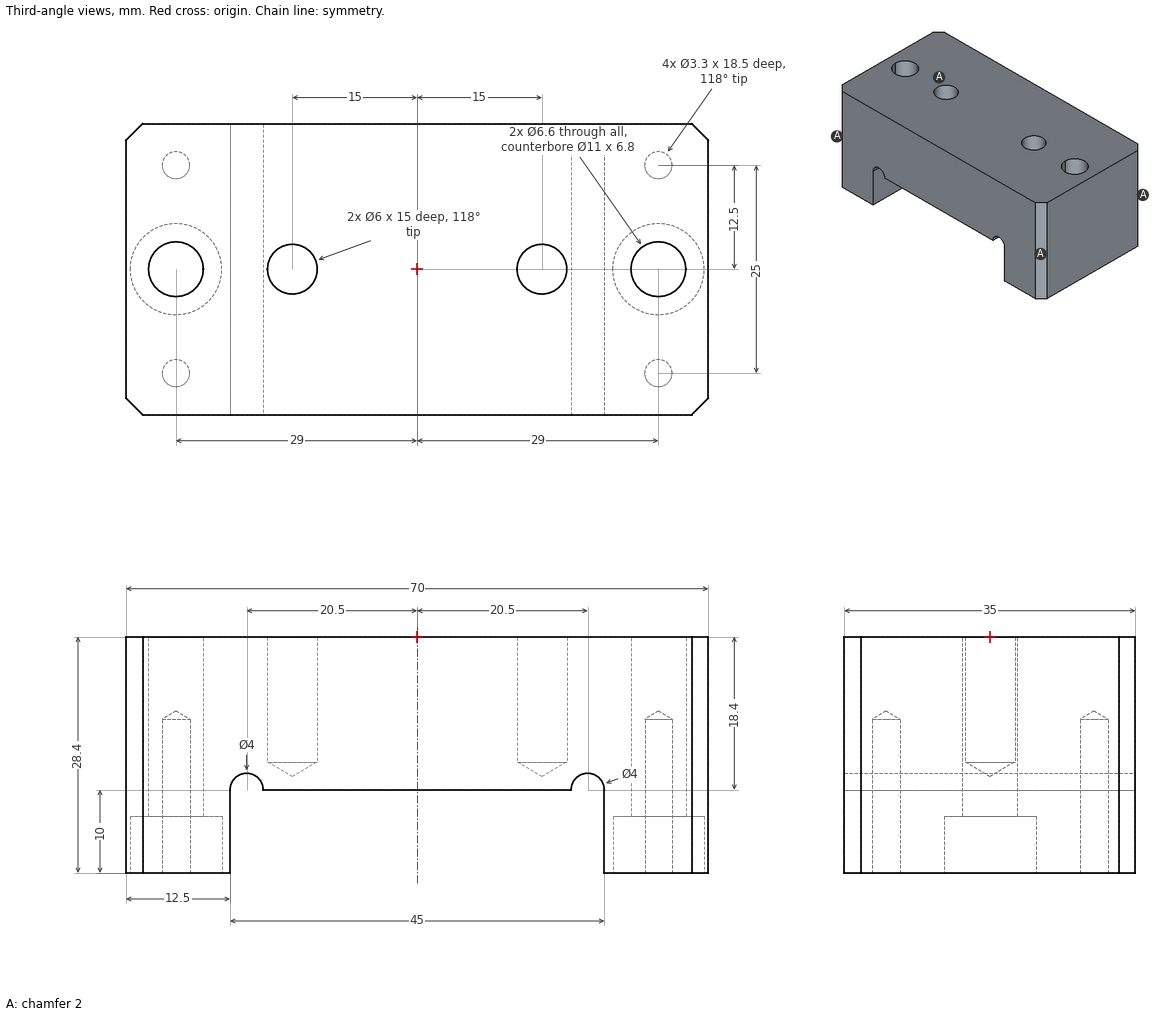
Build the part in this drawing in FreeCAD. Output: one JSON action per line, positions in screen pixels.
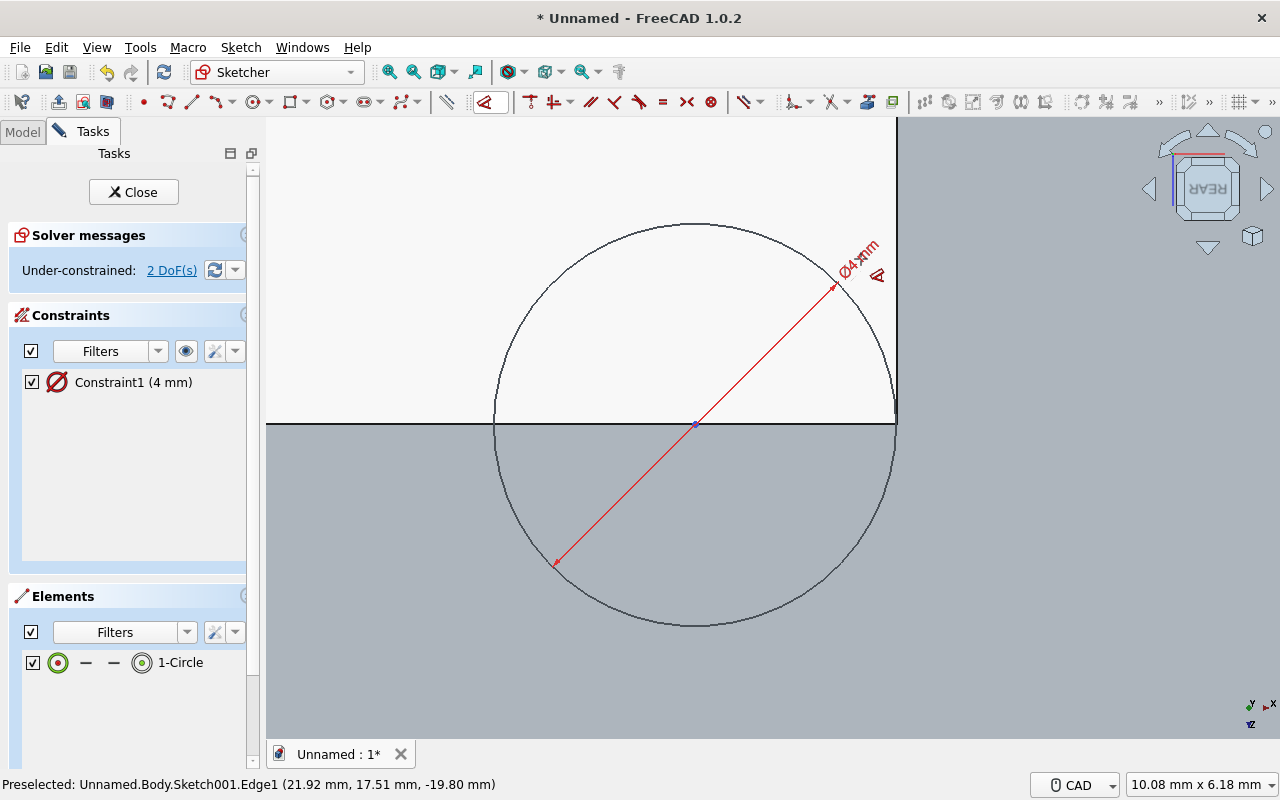
{"action": "left_click", "coordinate": [695, 425]}
{"action": "left_click", "coordinate": [402, 391]}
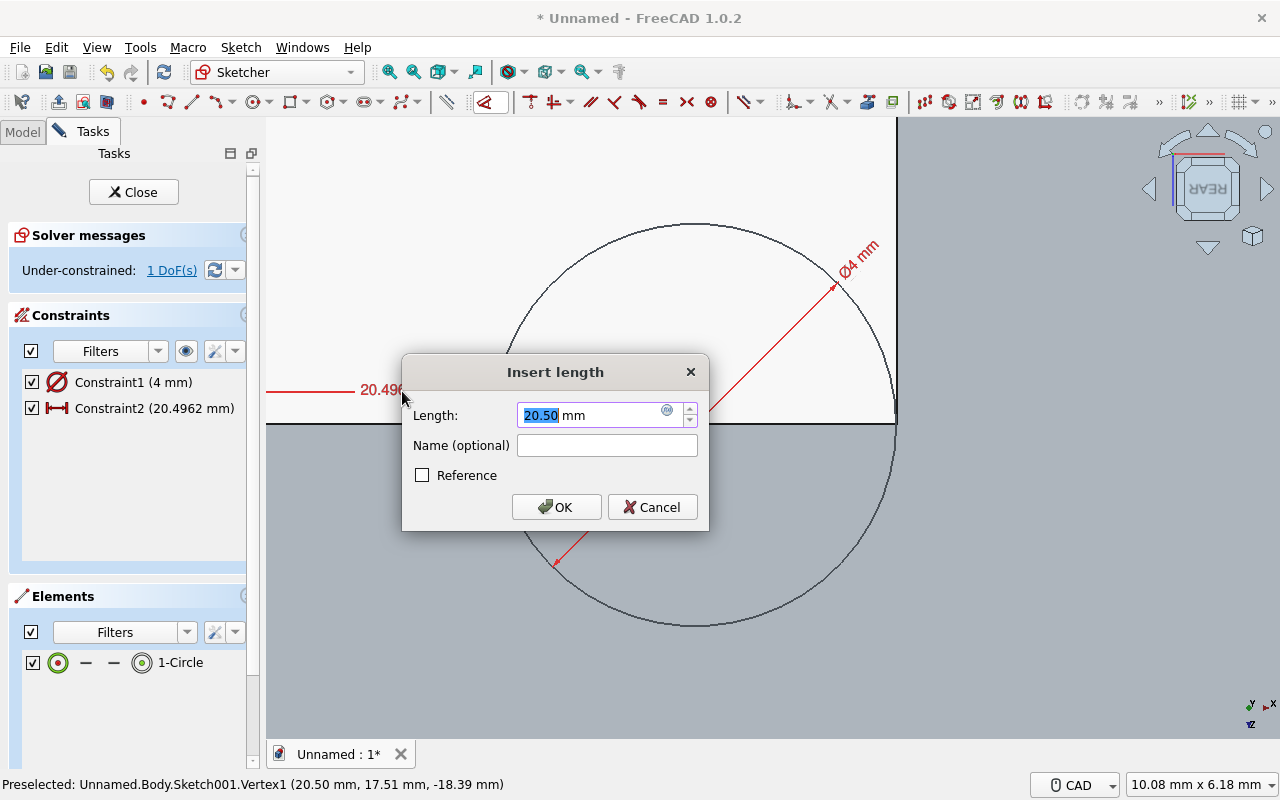
{"action": "type", "text": "20.5"}
{"action": "key", "text": "Return"}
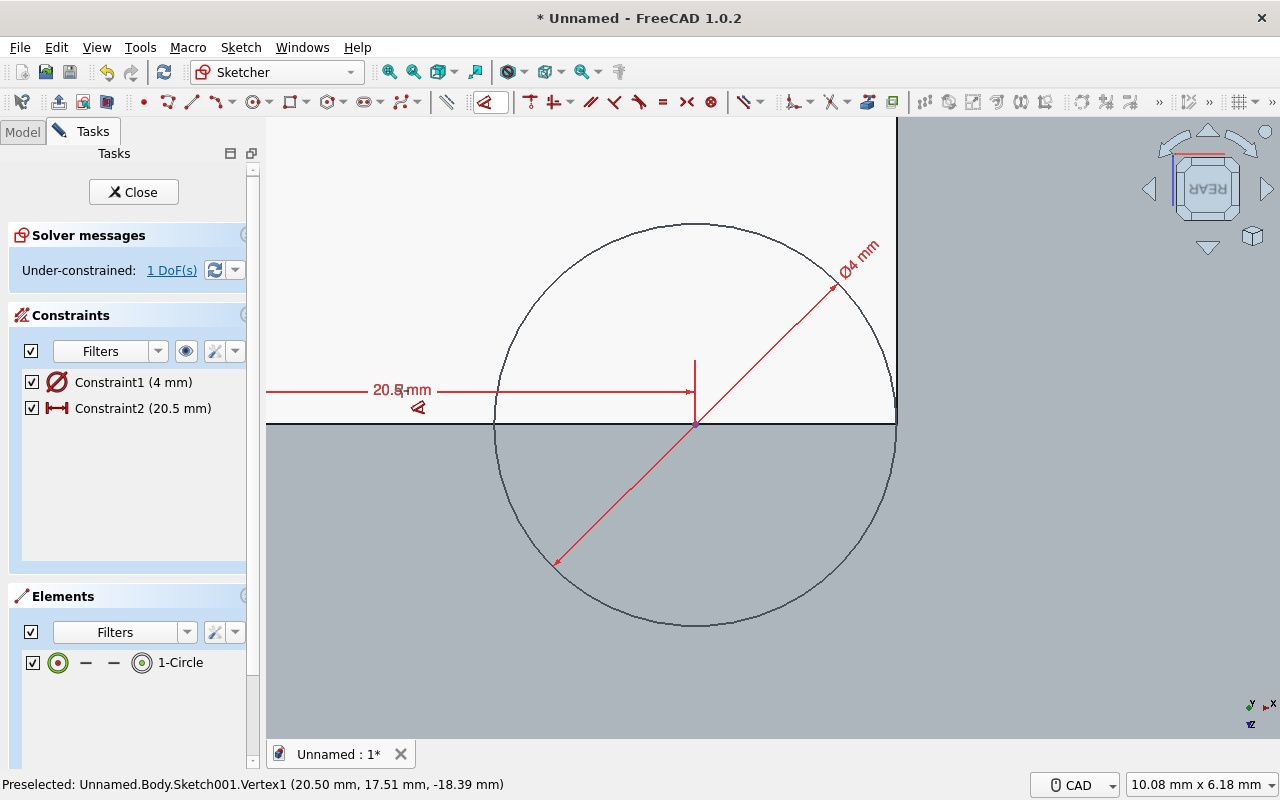
{"action": "left_click", "coordinate": [695, 425]}
{"action": "left_click", "coordinate": [729, 568]}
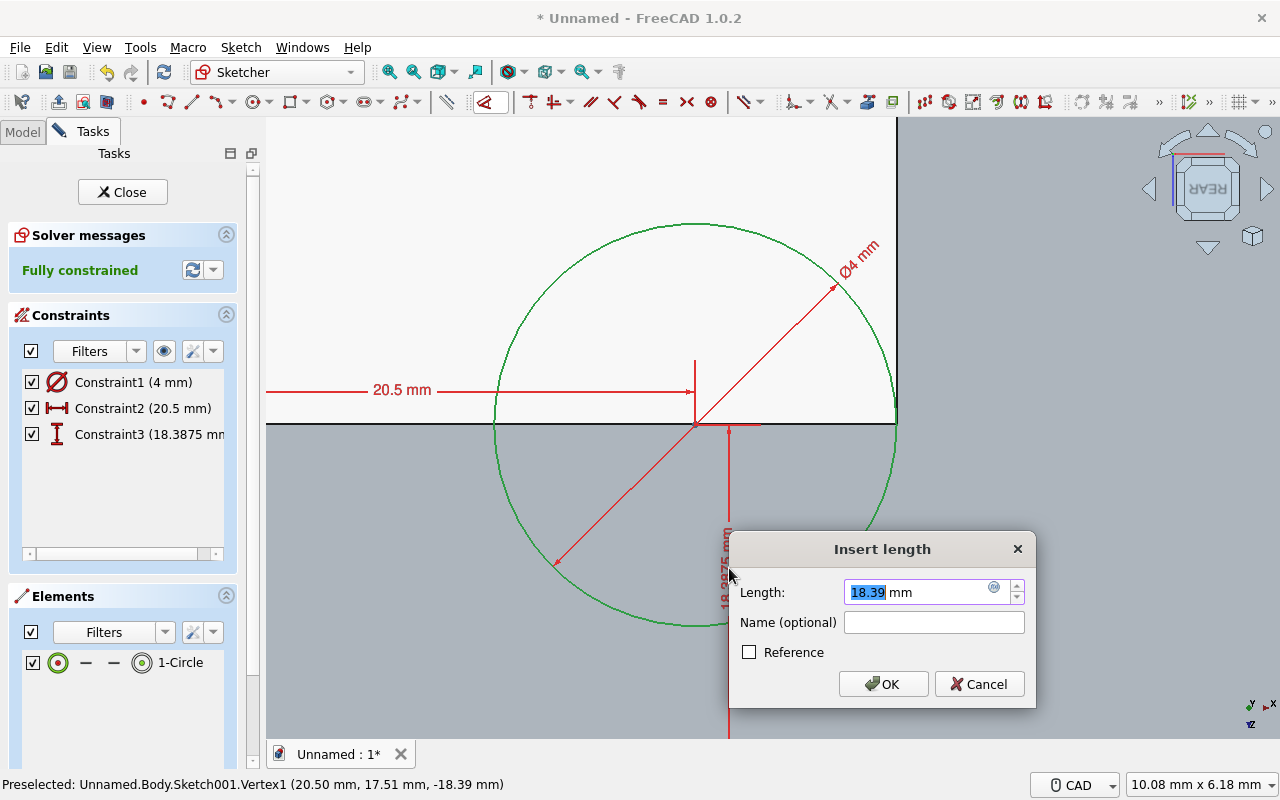
{"action": "type", "text": "18.4"}
{"action": "key", "text": "Return"}
{"action": "key", "text": "Escape"}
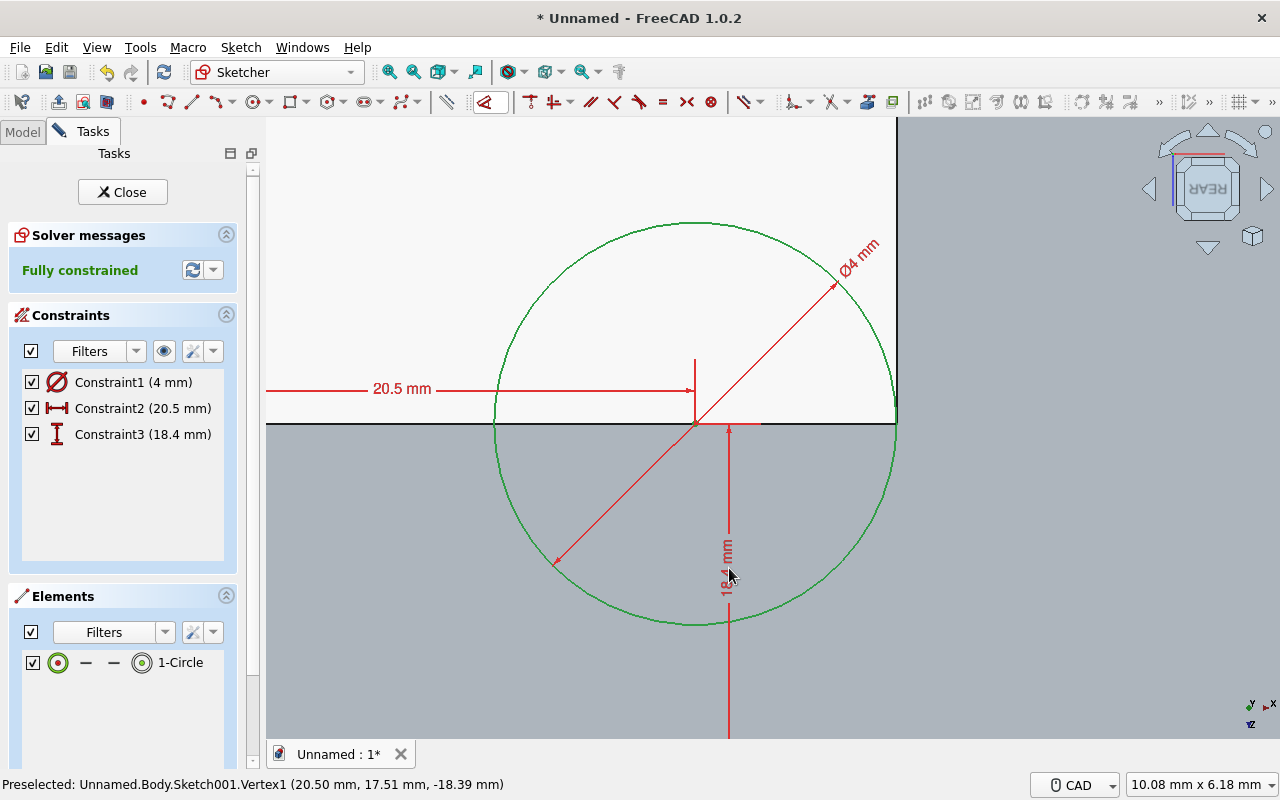
{"action": "left_click", "coordinate": [123, 192]}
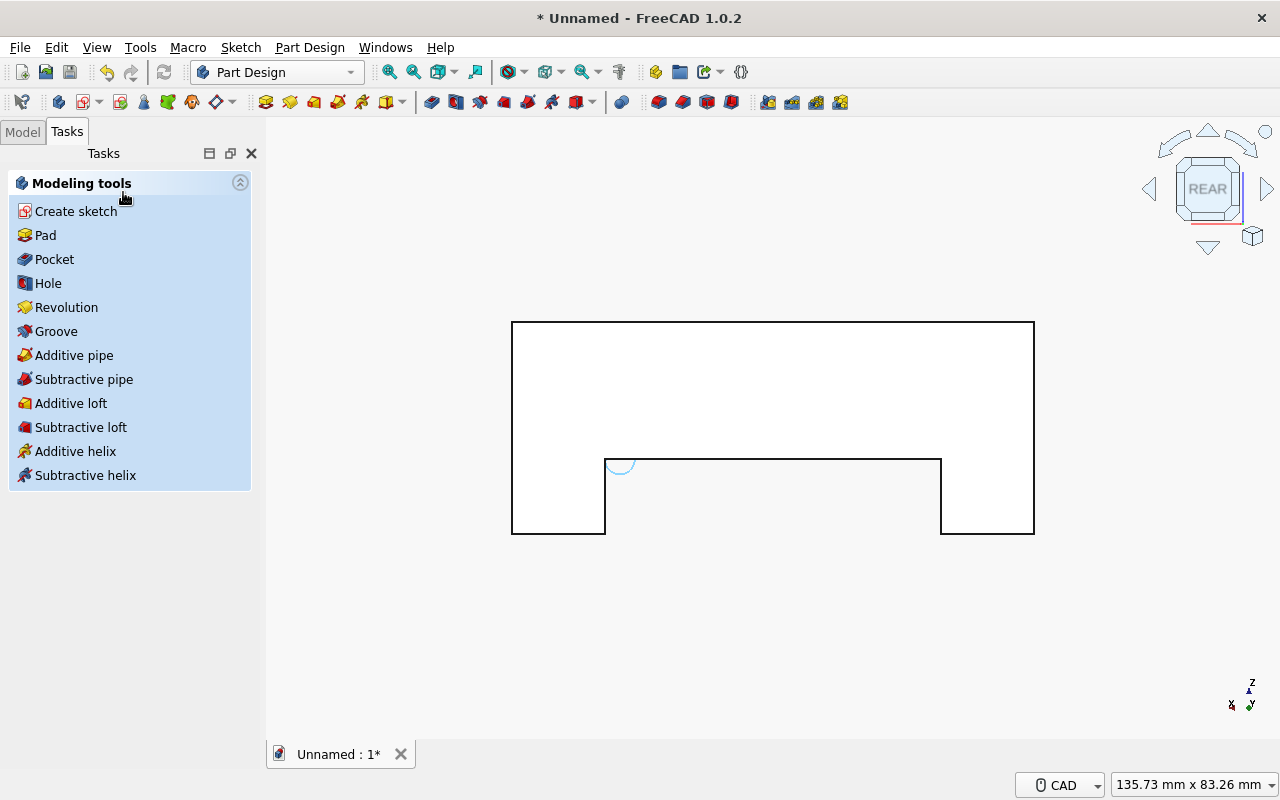
{"action": "left_click", "coordinate": [432, 102]}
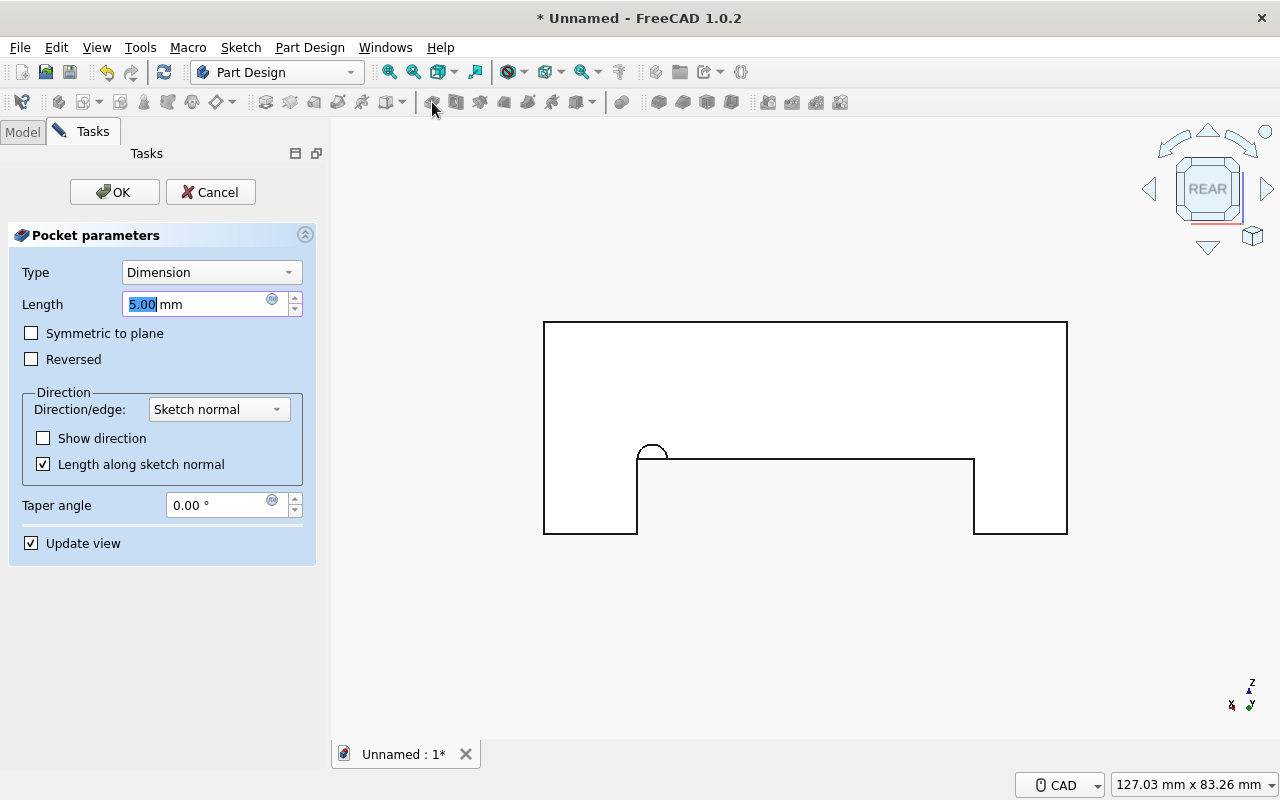
{"action": "left_click", "coordinate": [212, 272]}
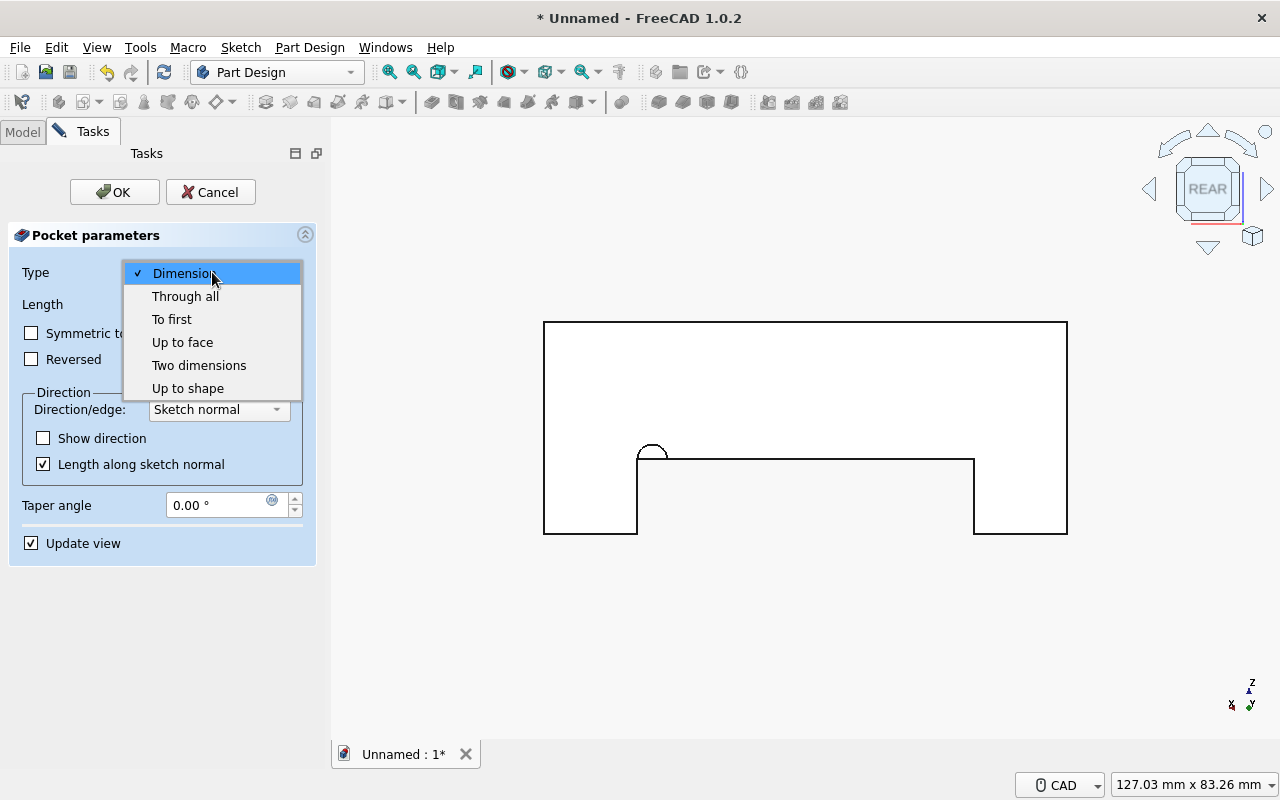
{"action": "left_click", "coordinate": [212, 320]}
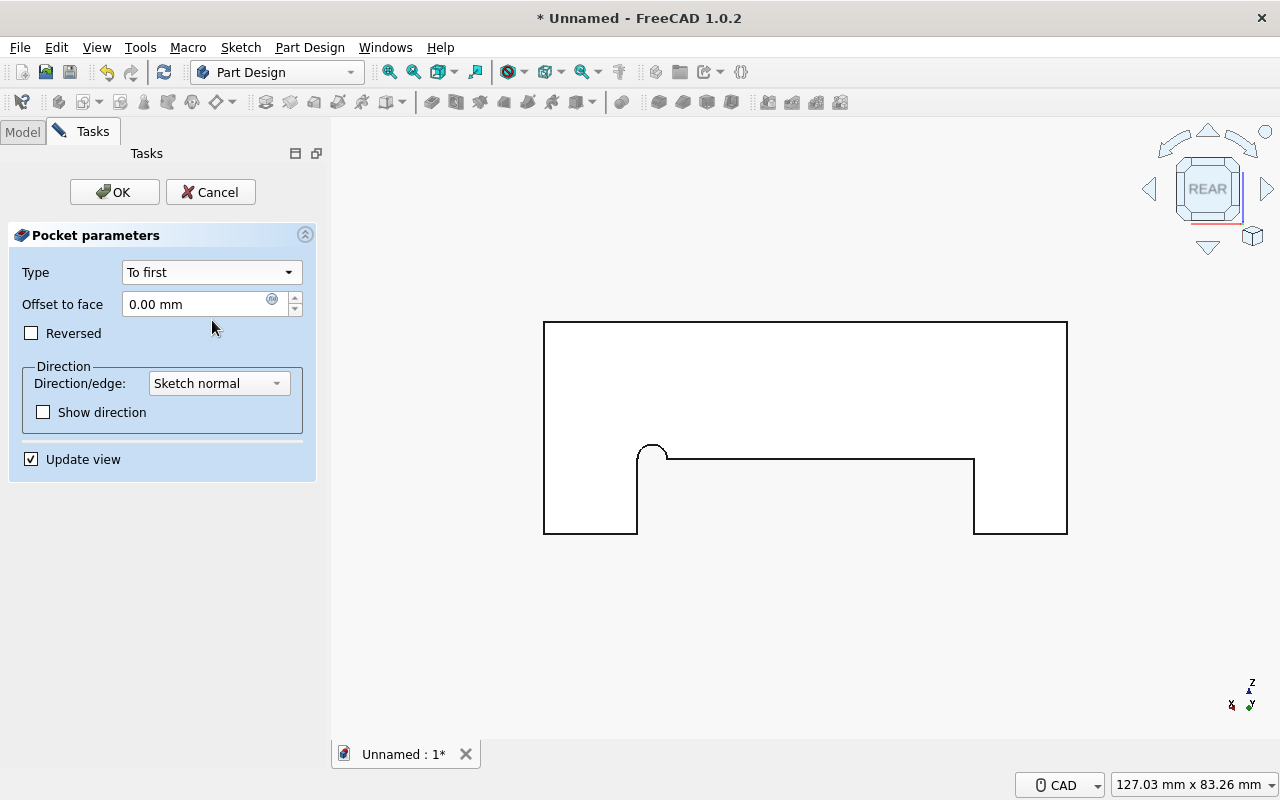
{"action": "left_click", "coordinate": [115, 192]}